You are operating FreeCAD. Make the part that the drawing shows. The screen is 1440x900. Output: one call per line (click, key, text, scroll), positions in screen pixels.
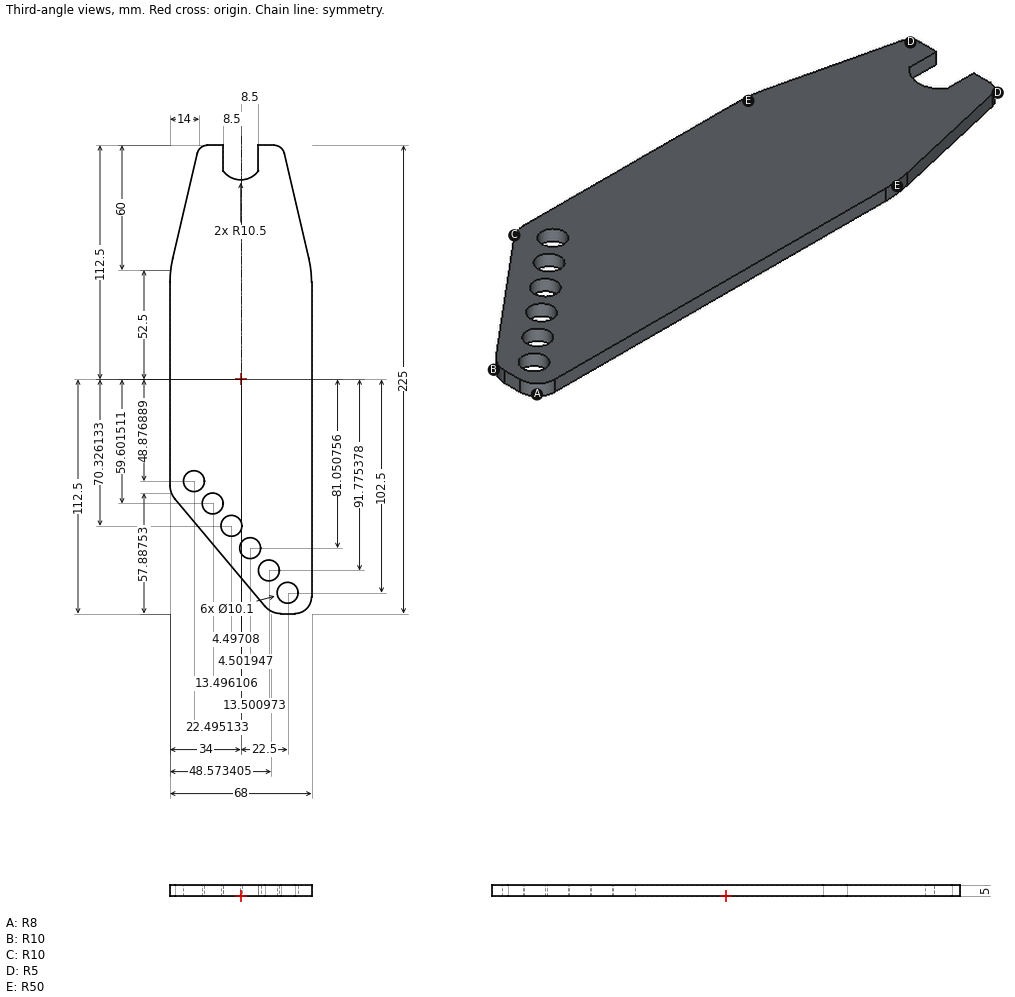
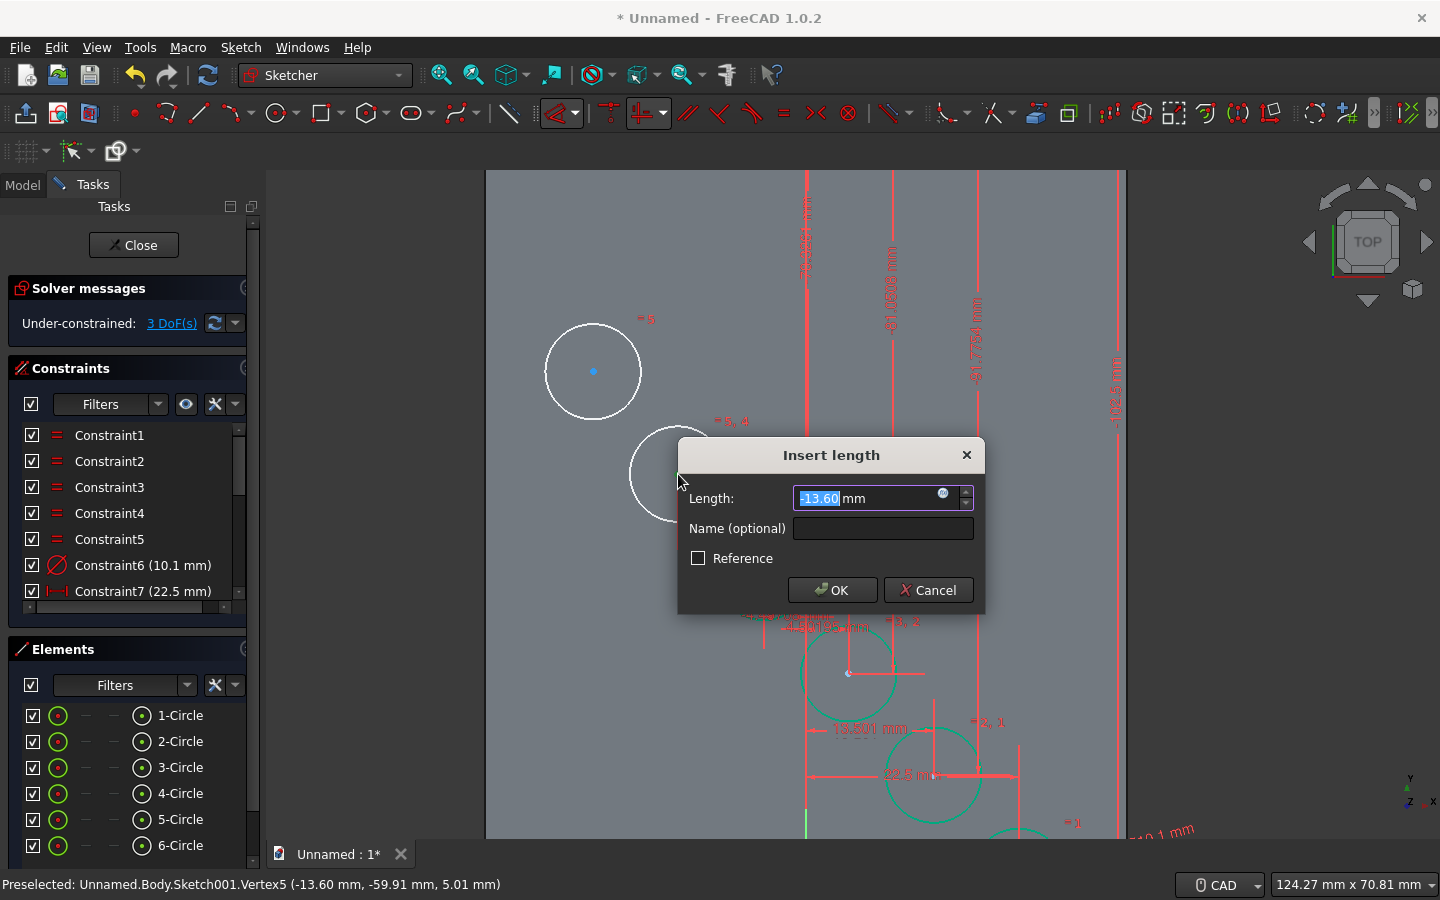
text(-13.496106)
key(Return)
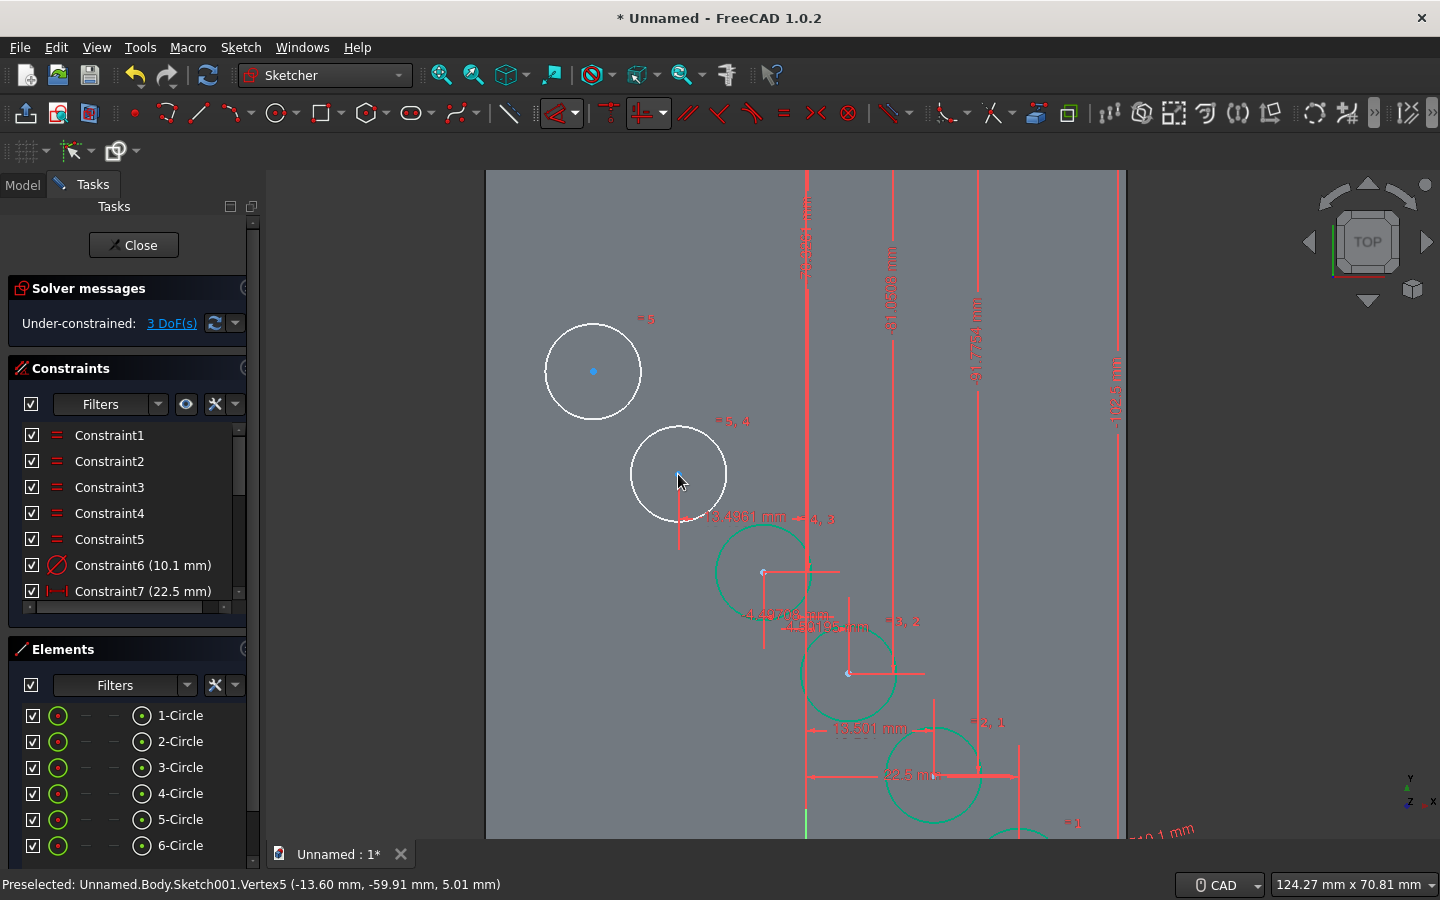
click(679, 474)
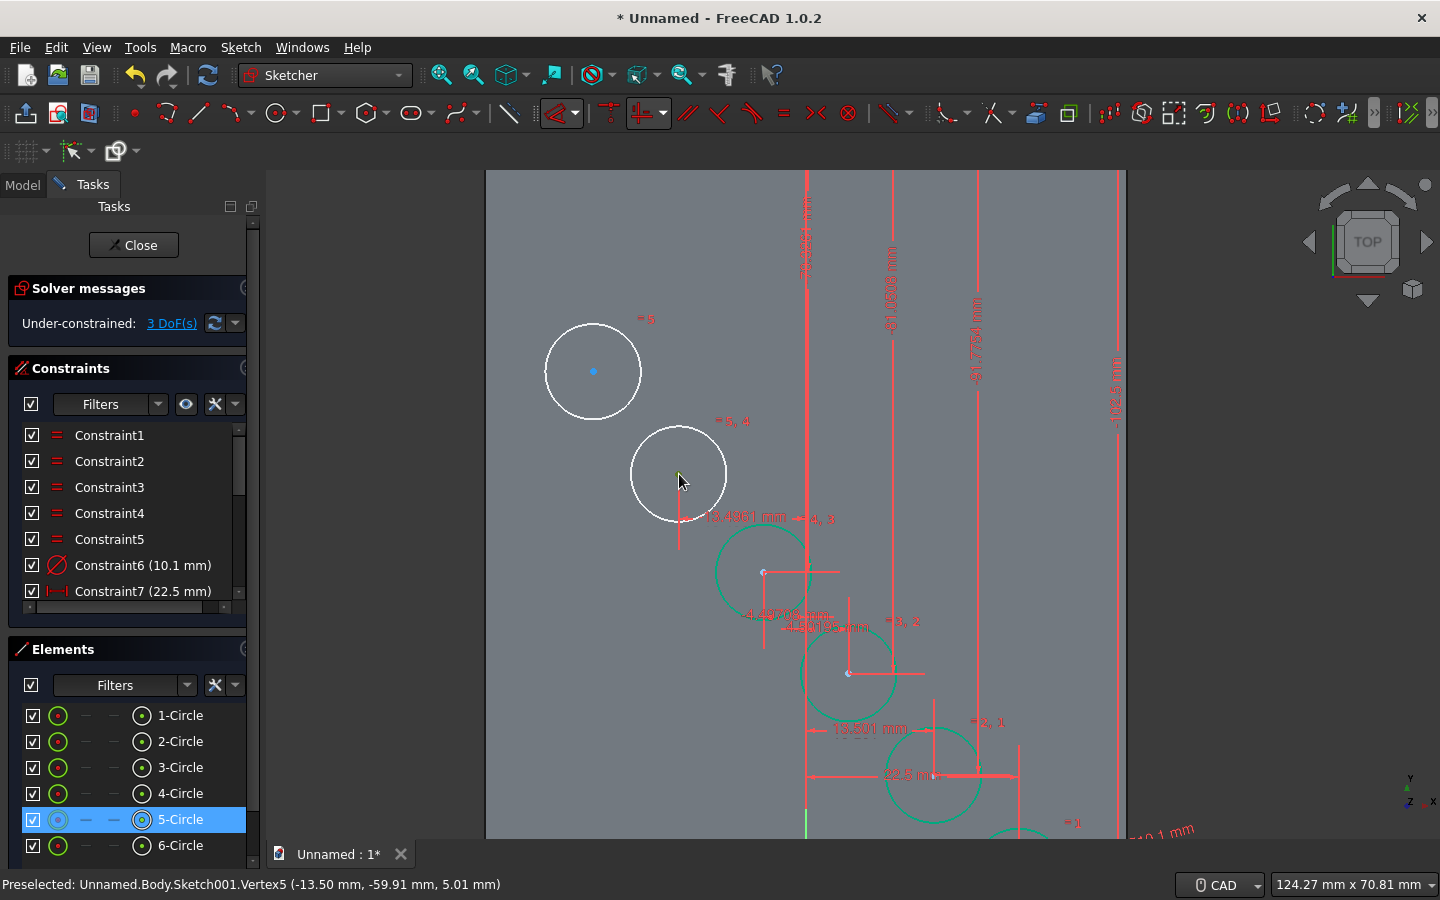
key(i)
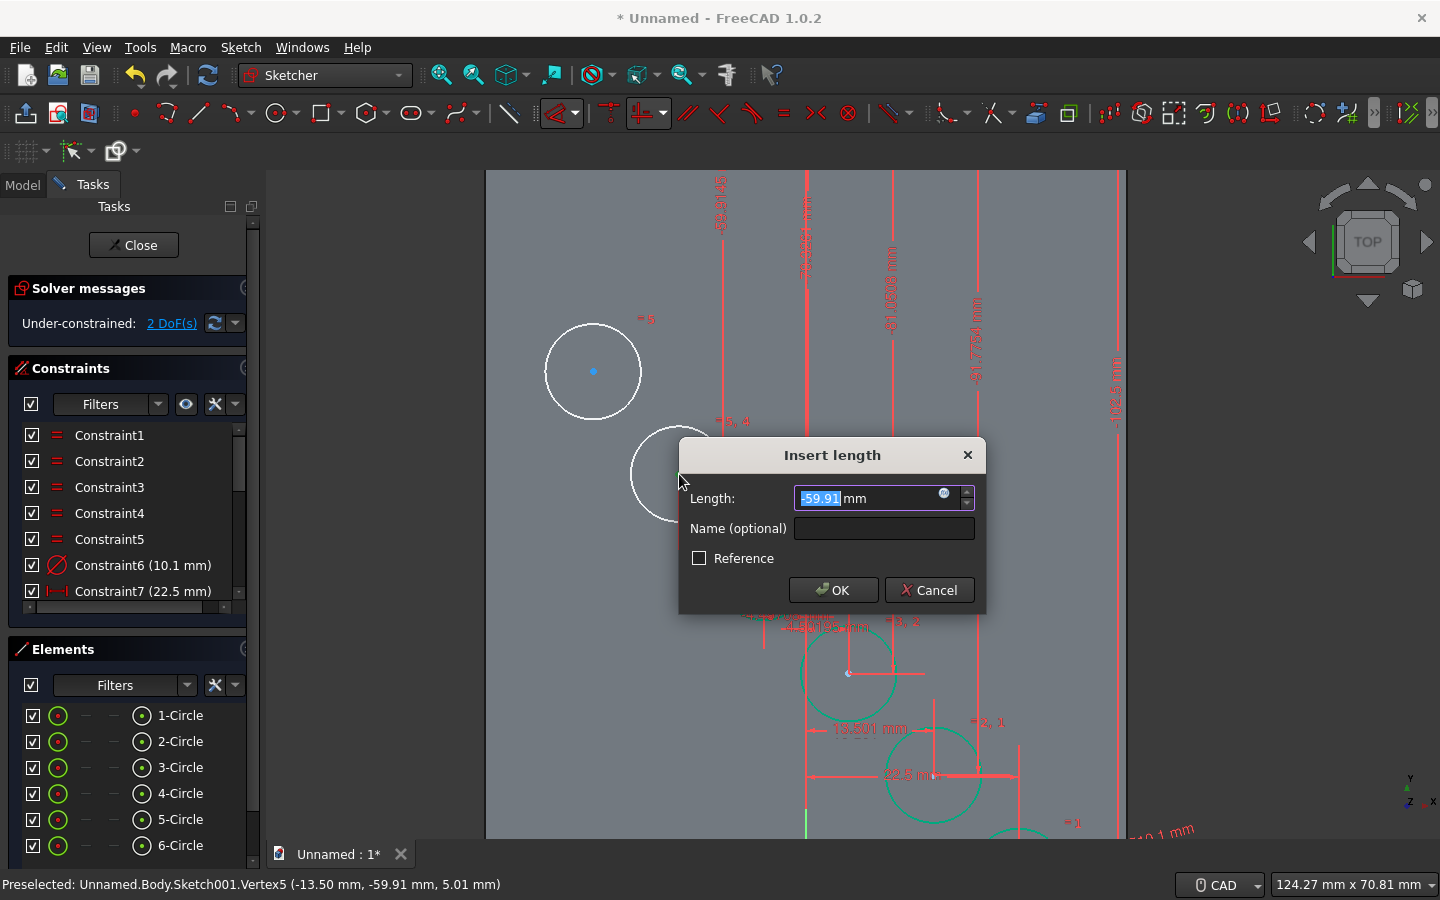
text(-59.601511)
key(Return)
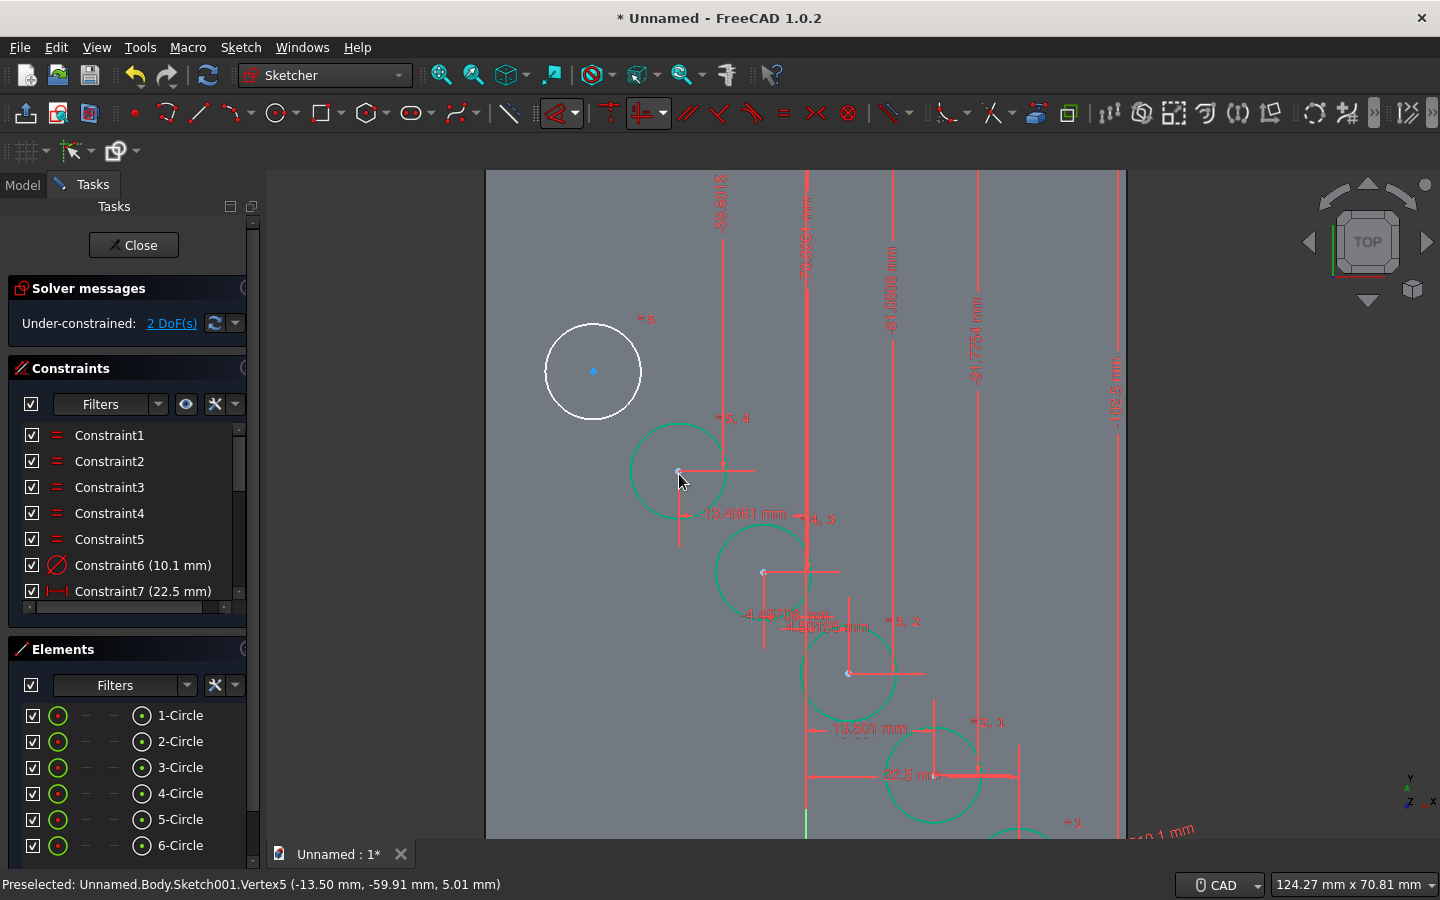
click(593, 372)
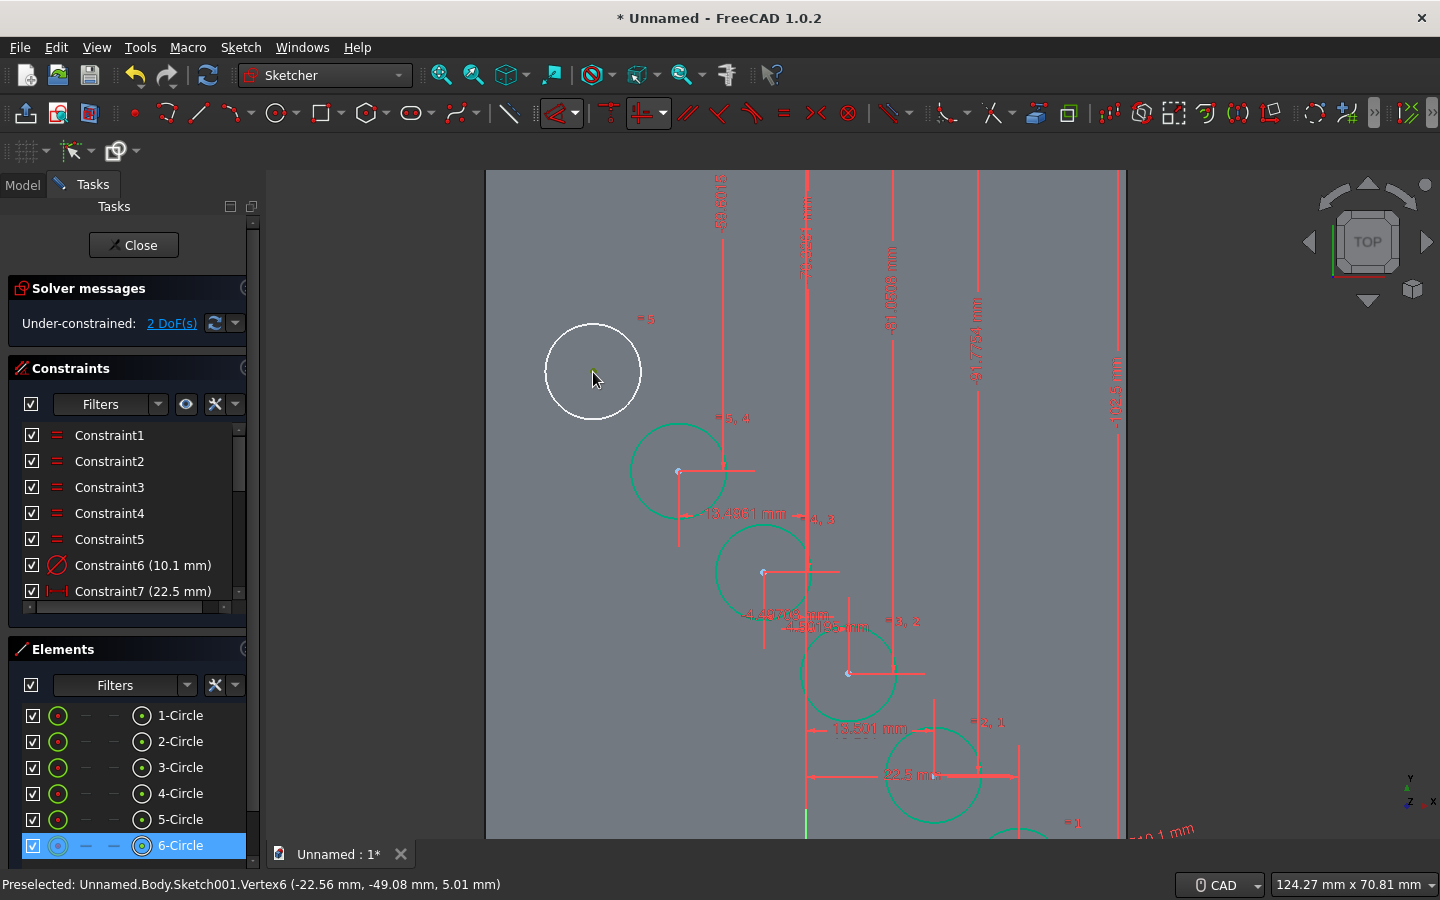
key(l)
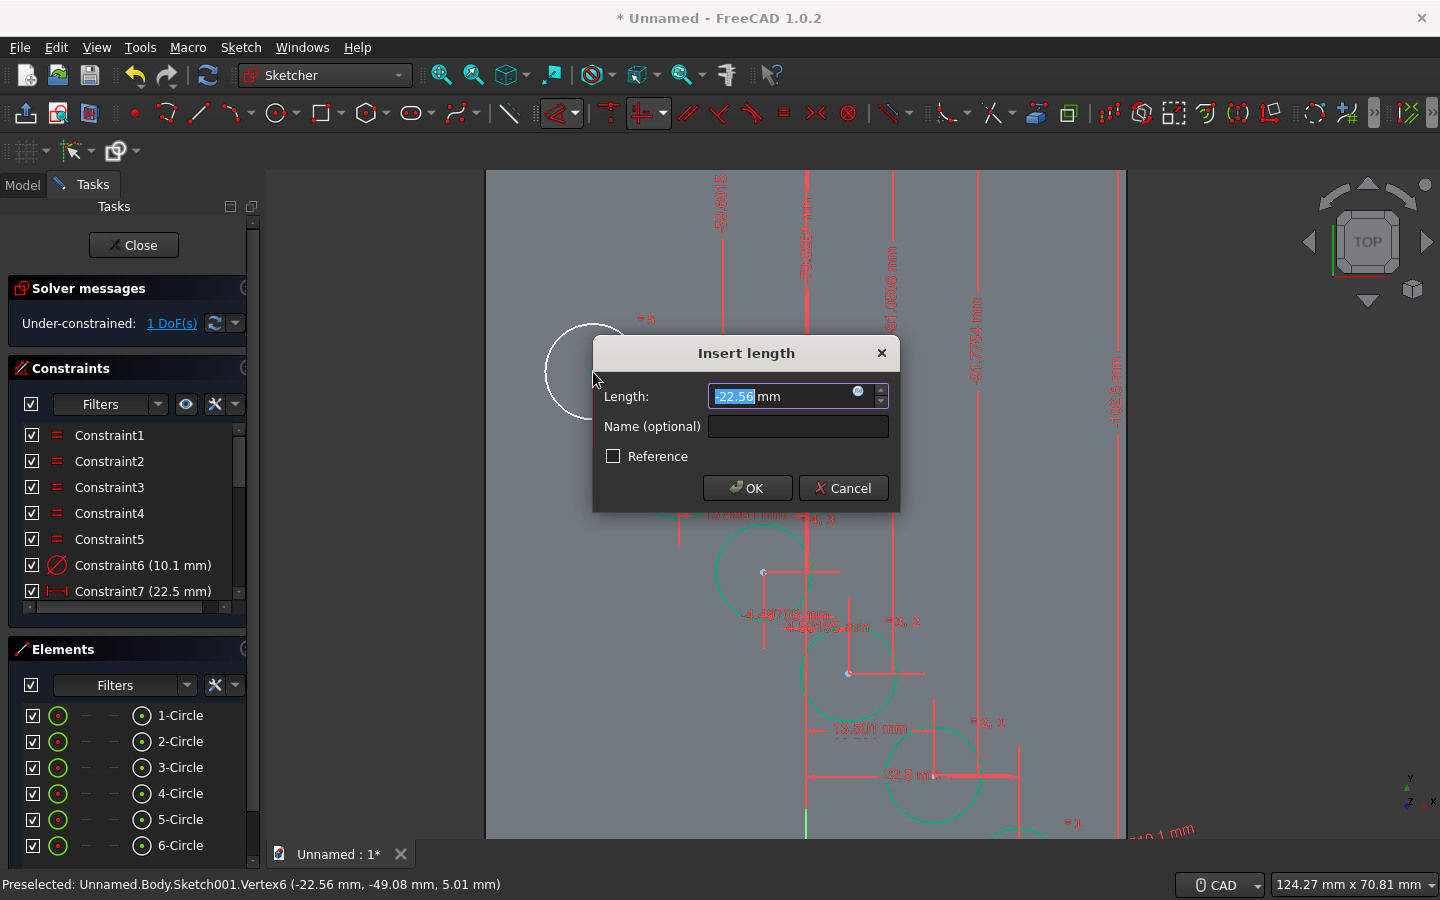
text(-22.495133)
key(Return)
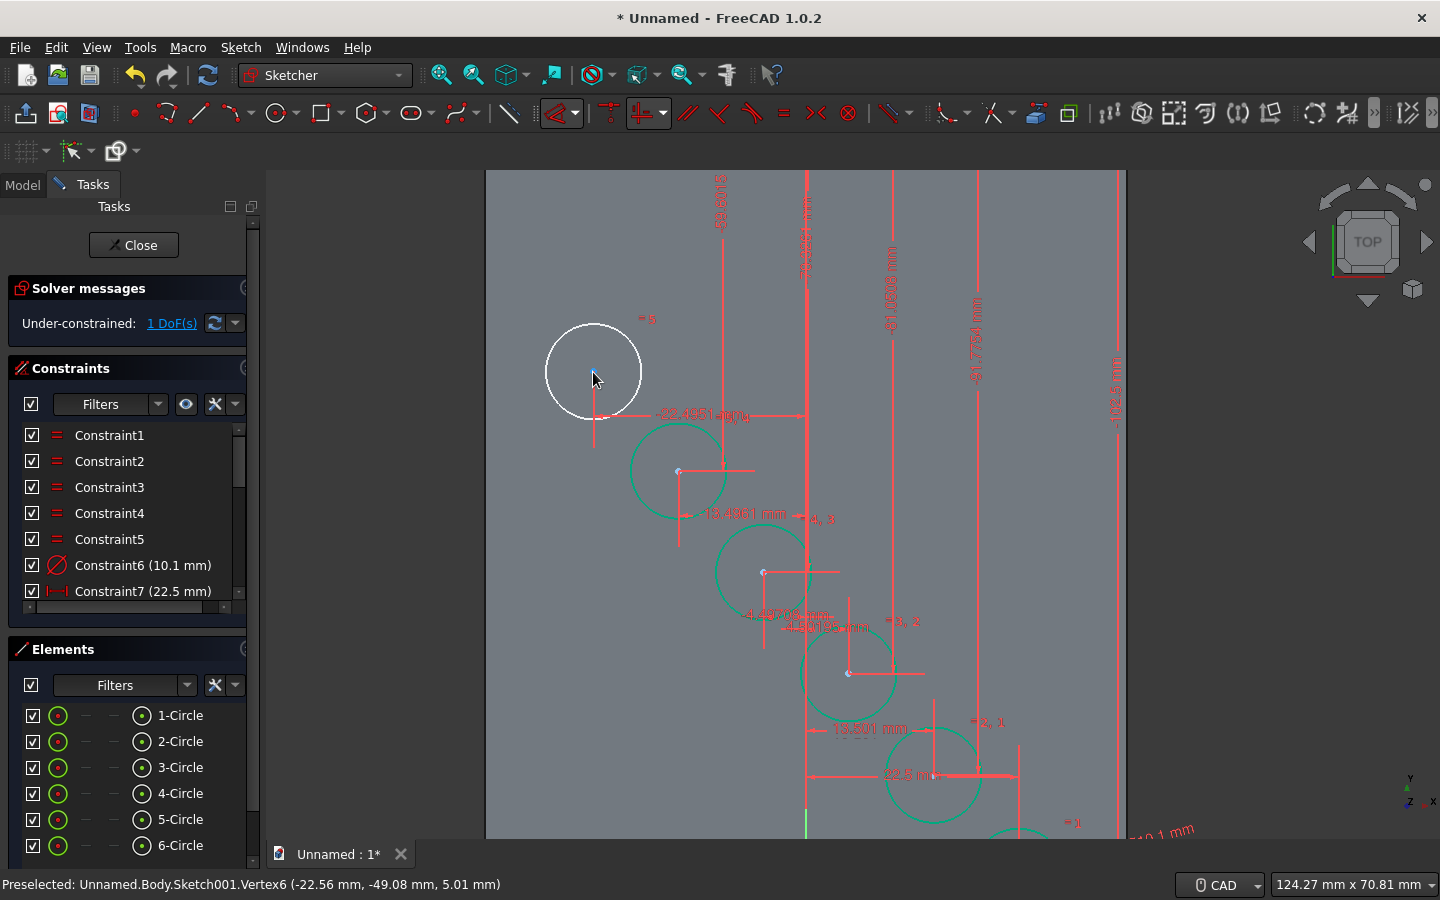
click(594, 372)